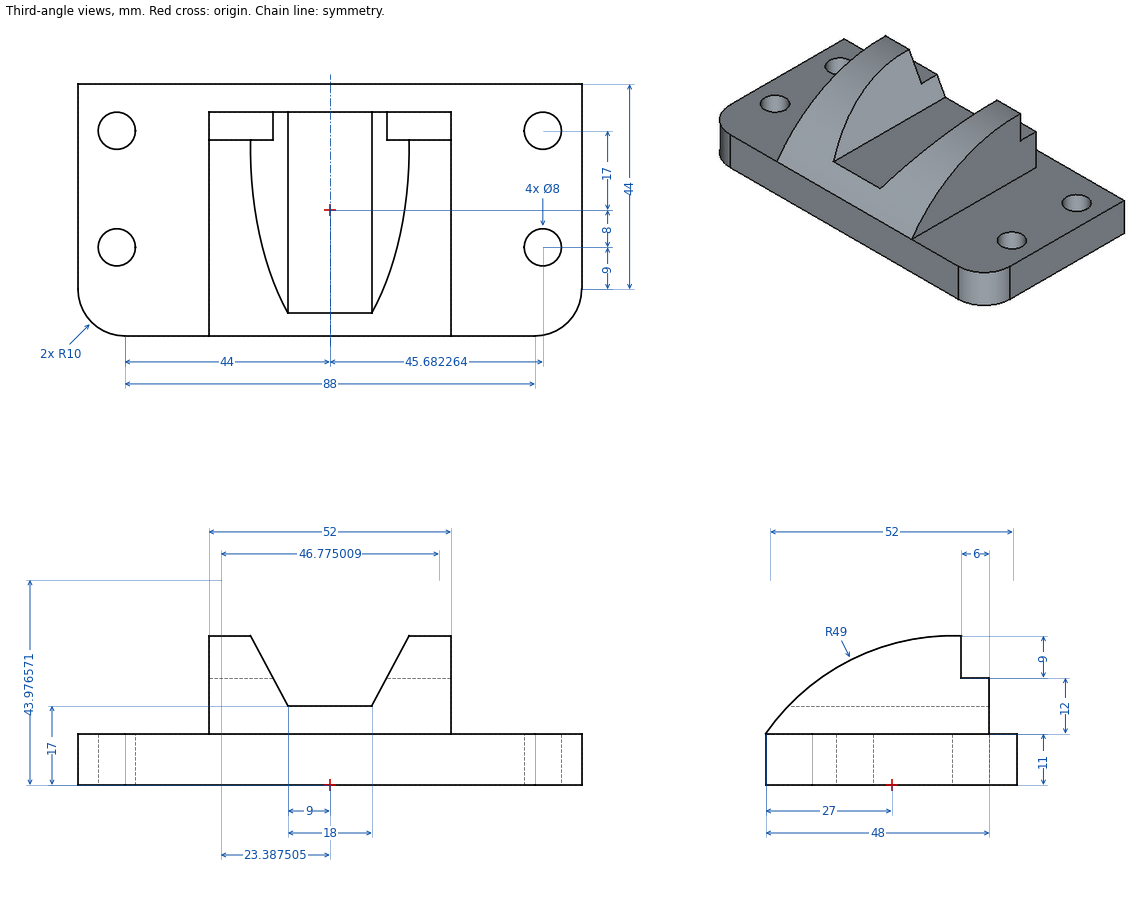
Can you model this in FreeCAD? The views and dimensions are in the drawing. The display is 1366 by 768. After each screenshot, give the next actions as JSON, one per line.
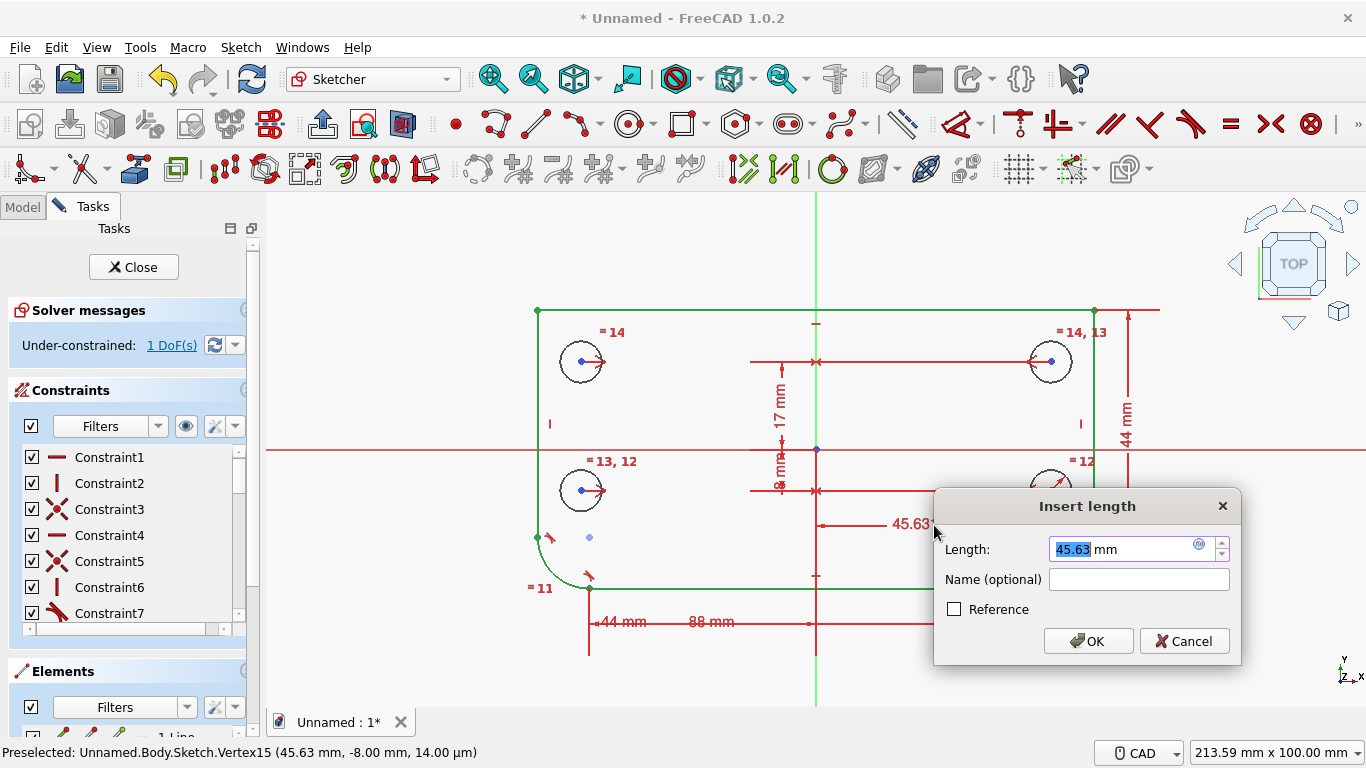
{"action": "type", "text": "45.682264"}
{"action": "key", "text": "Return"}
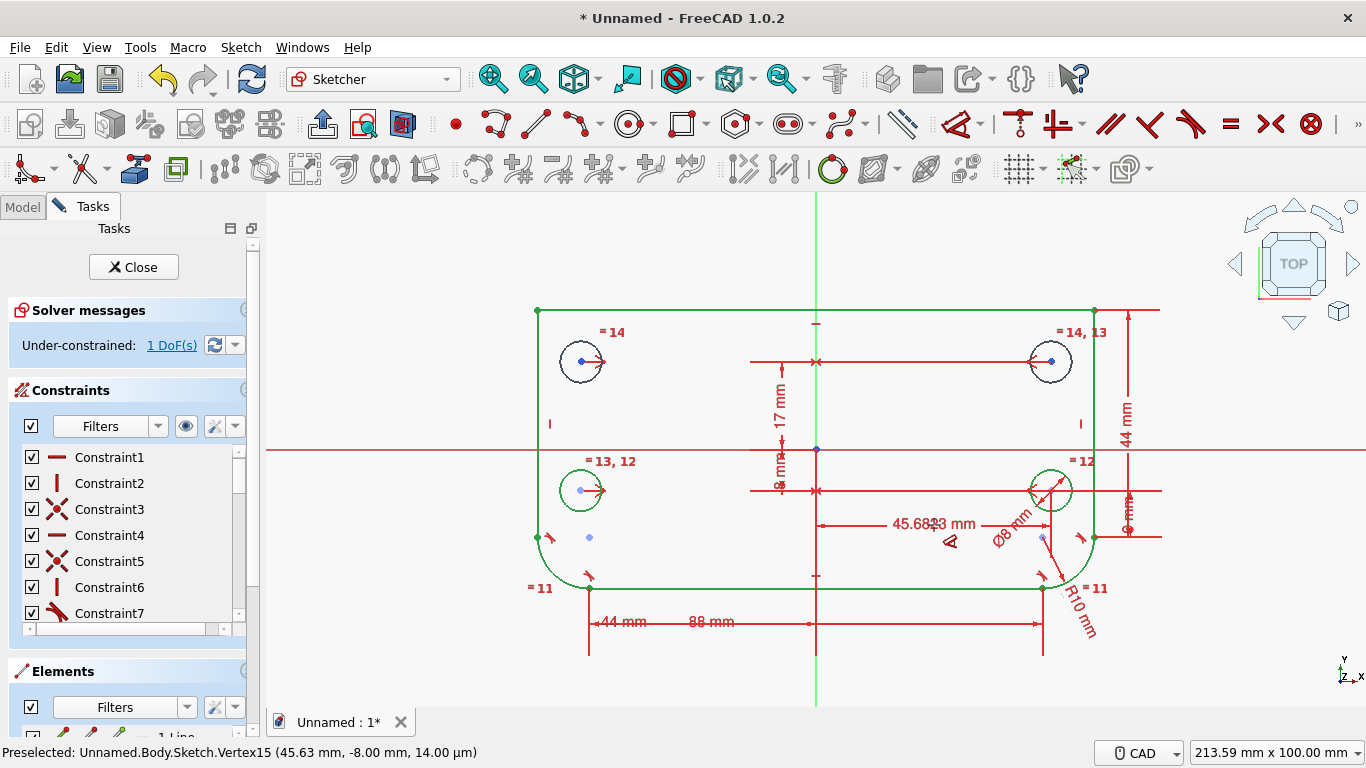
{"action": "left_click", "coordinate": [1051, 362]}
{"action": "left_click", "coordinate": [934, 328]}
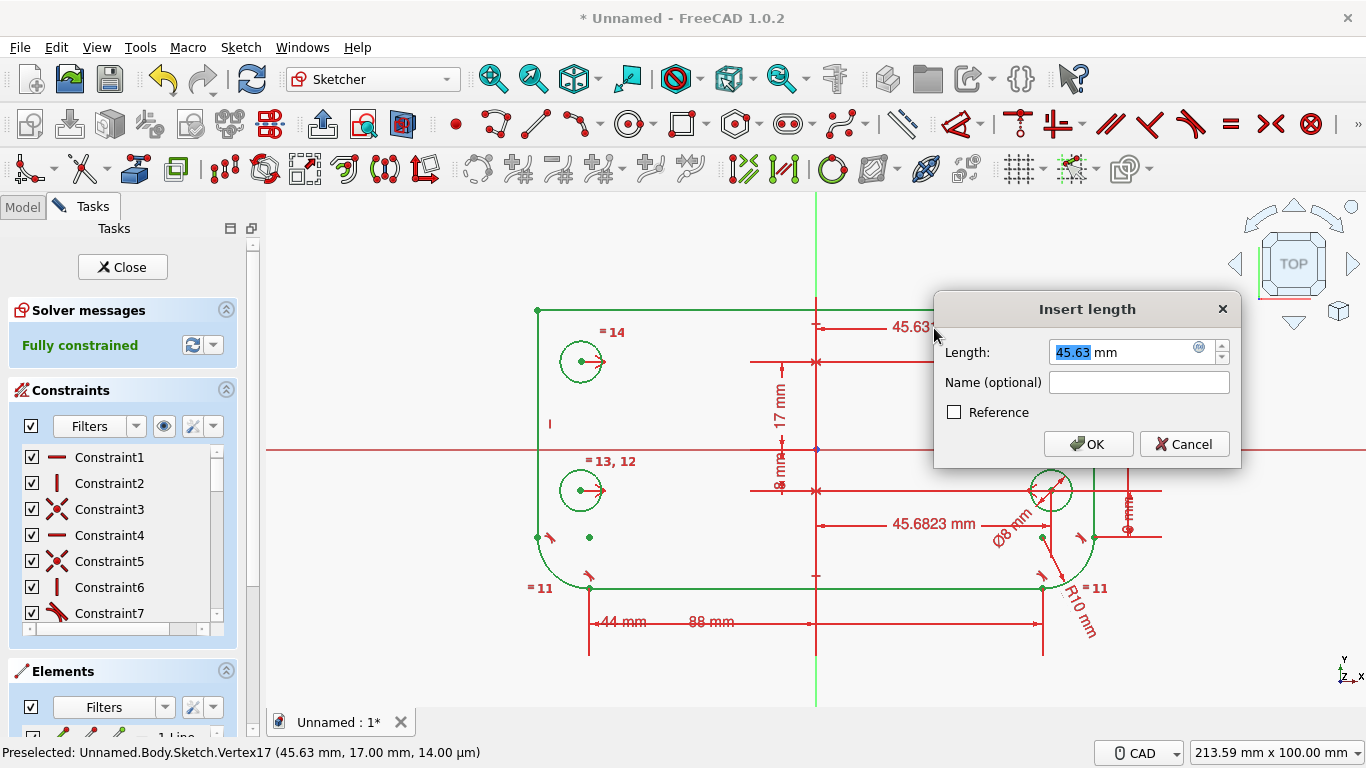
{"action": "type", "text": "45.682264"}
{"action": "key", "text": "Return"}
{"action": "key", "text": "Escape"}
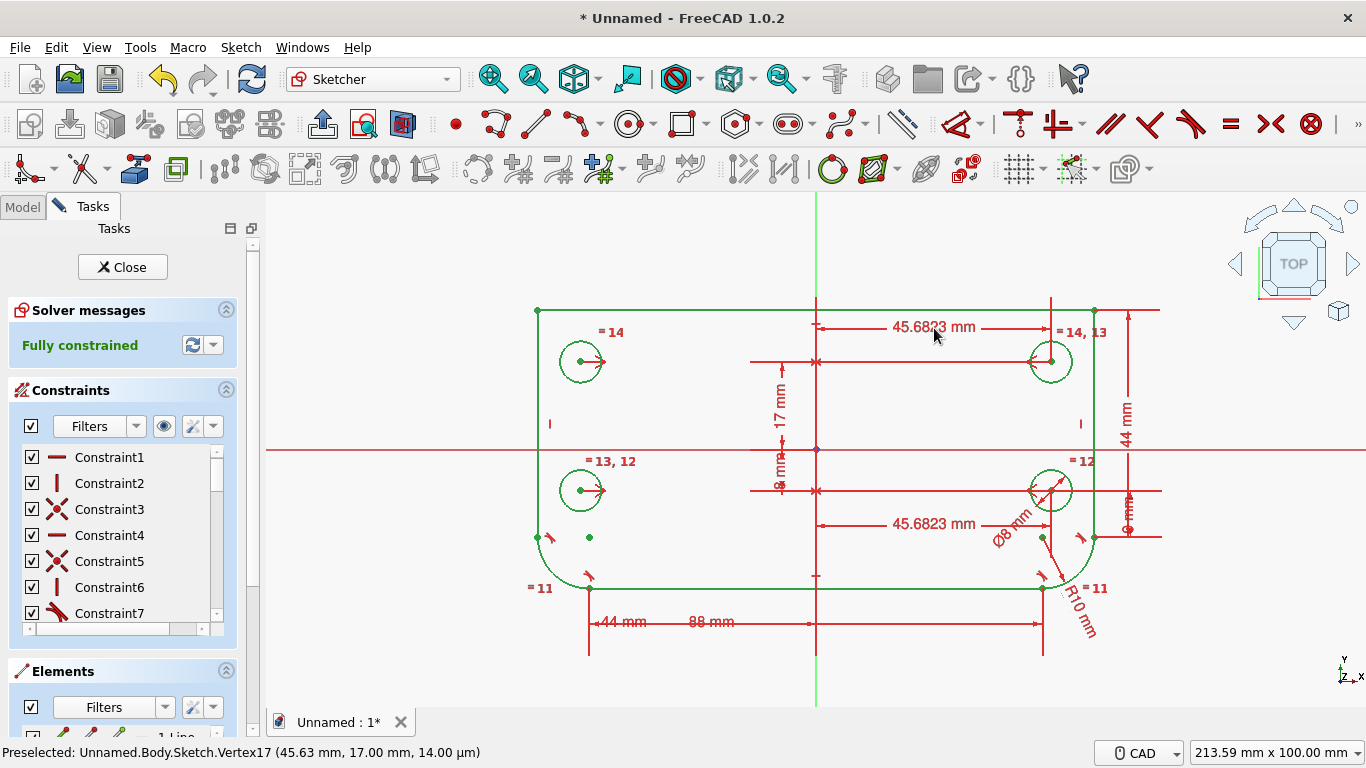
{"action": "left_click", "coordinate": [123, 267]}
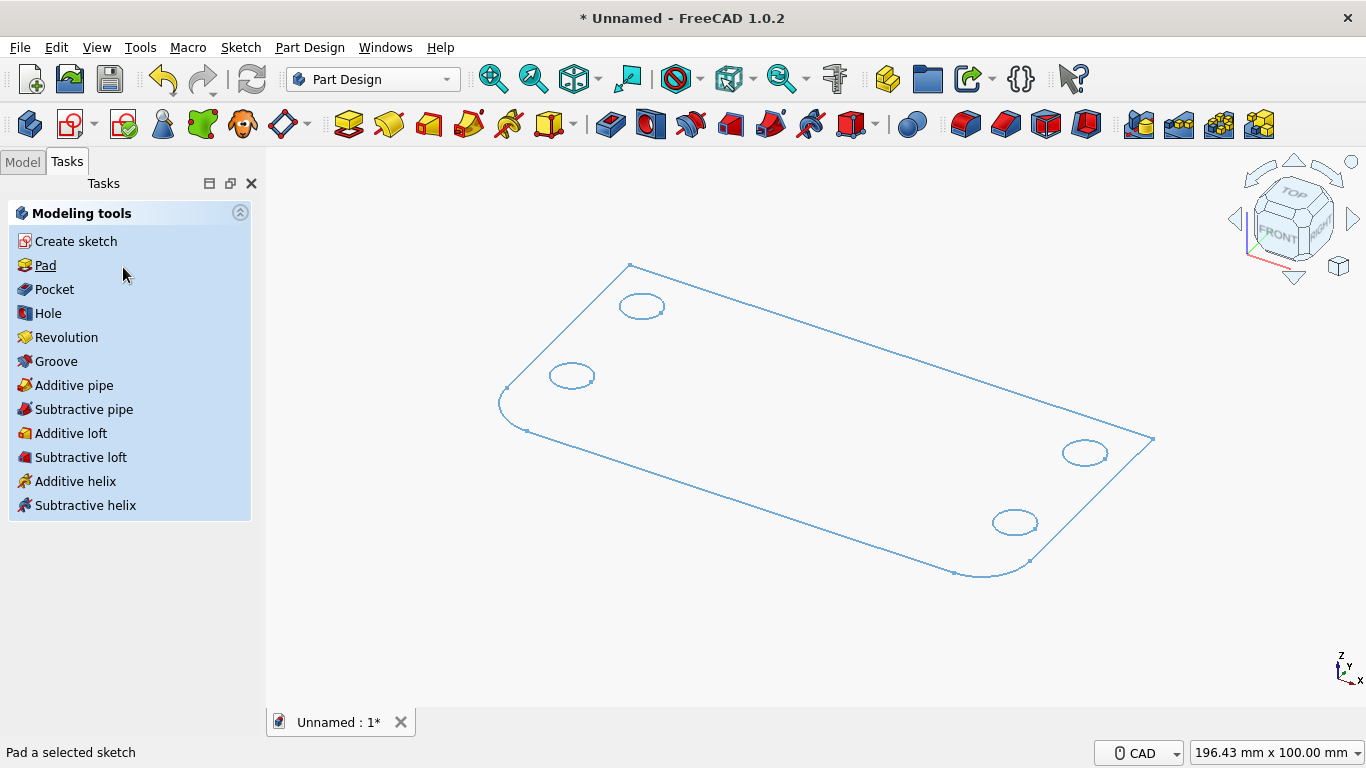
{"action": "left_click", "coordinate": [350, 124]}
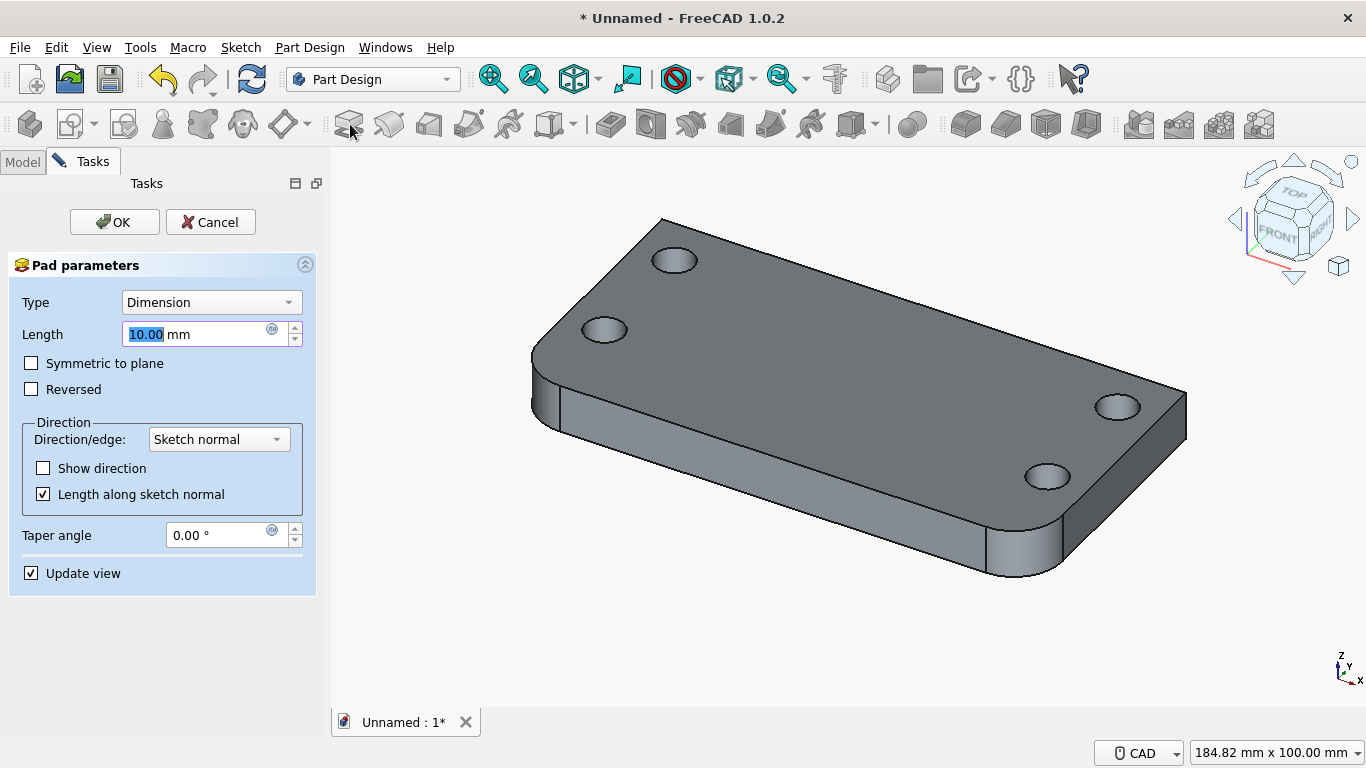
{"action": "type", "text": "11"}
{"action": "key", "text": "Tab"}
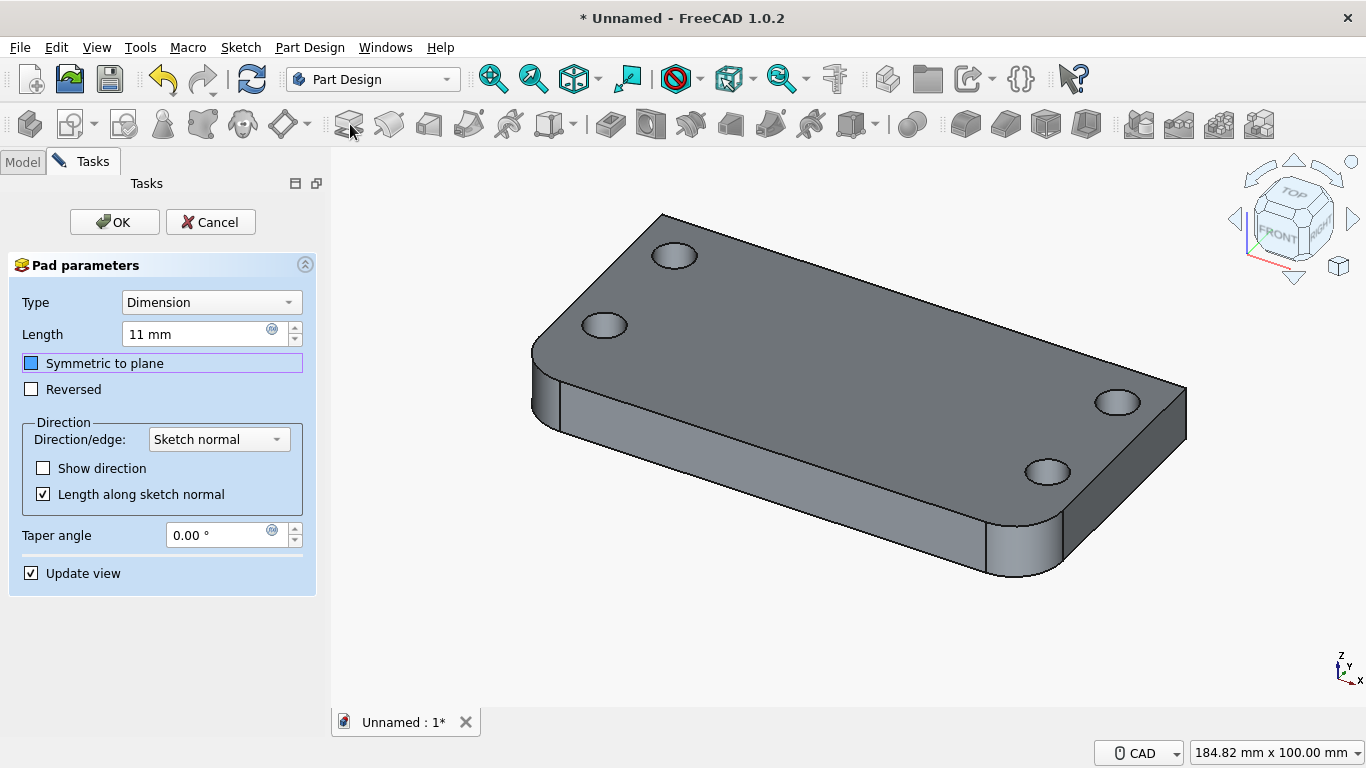
{"action": "left_click", "coordinate": [115, 222]}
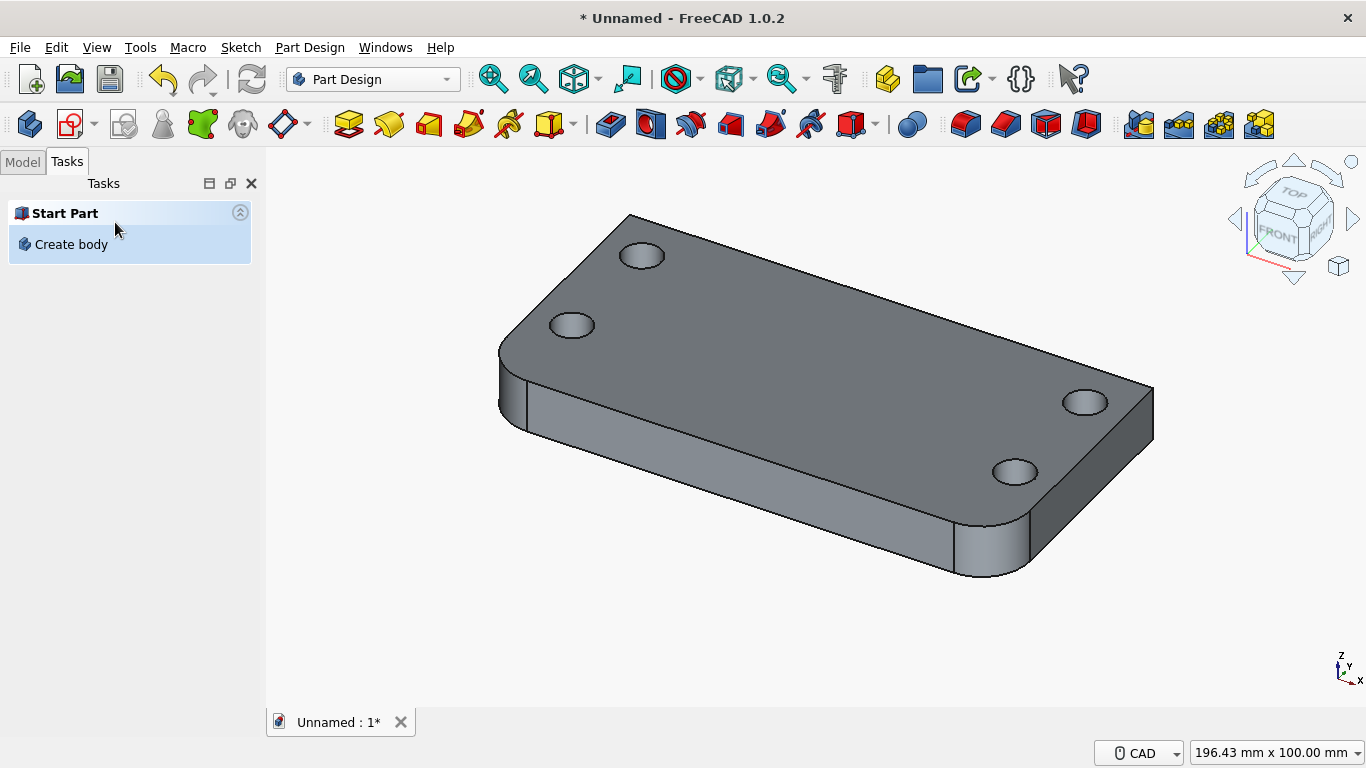
{"action": "left_click", "coordinate": [70, 124]}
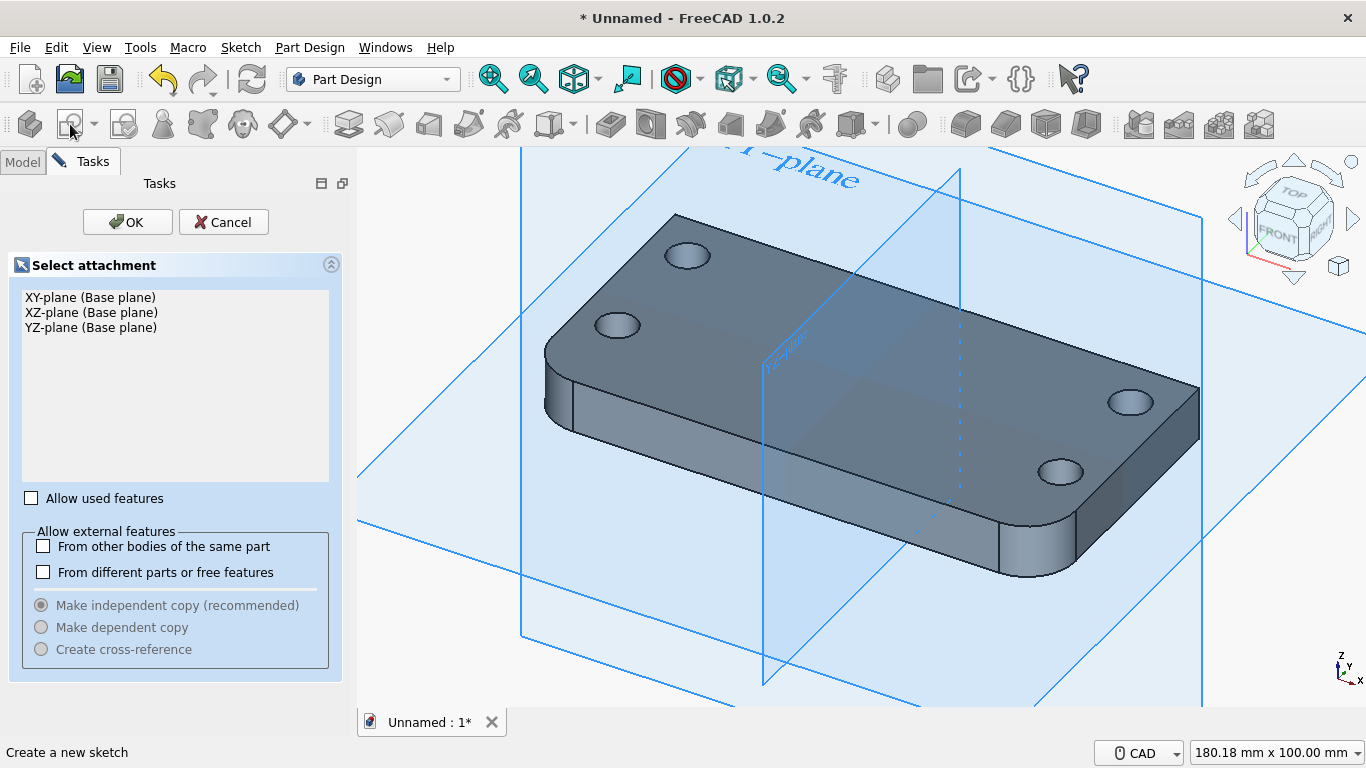
{"action": "left_click", "coordinate": [82, 328]}